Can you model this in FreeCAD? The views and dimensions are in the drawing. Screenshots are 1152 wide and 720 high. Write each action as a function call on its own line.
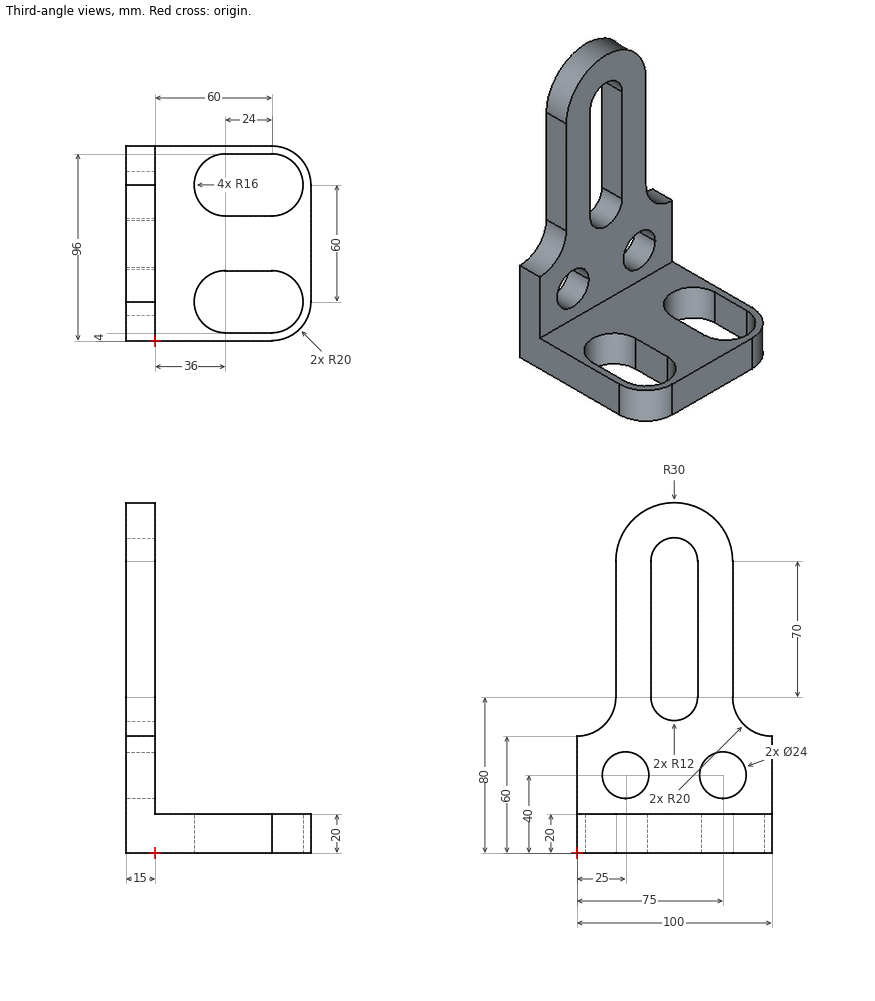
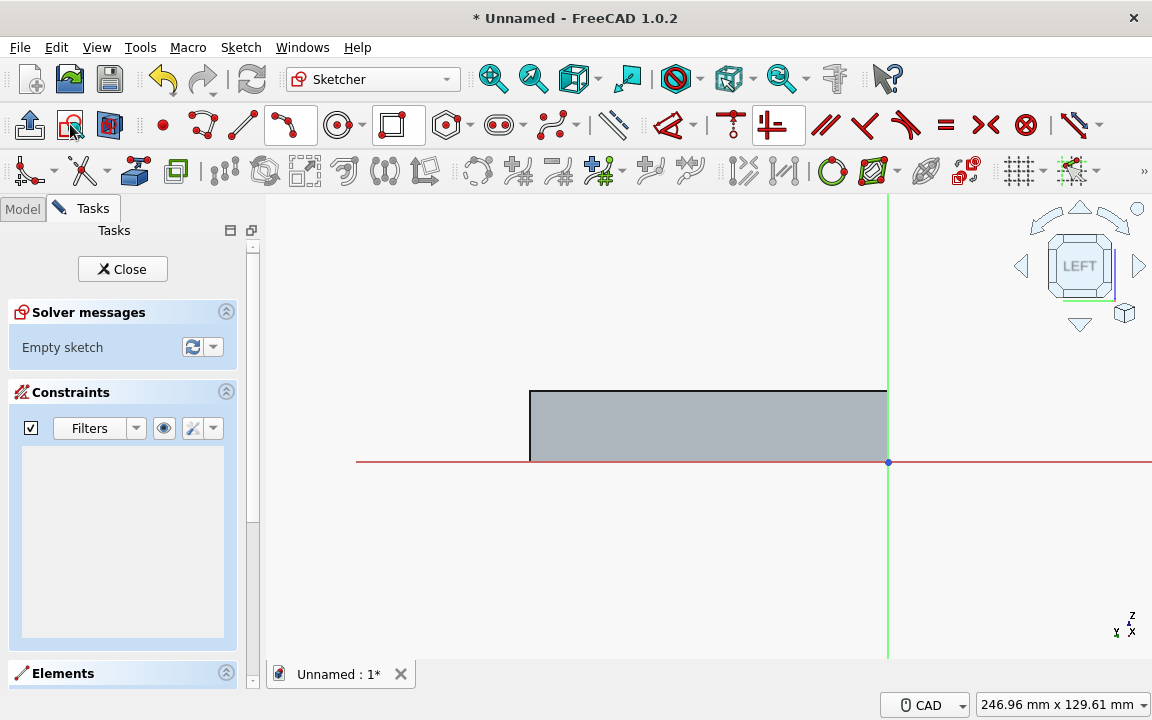
key(g)
key(r)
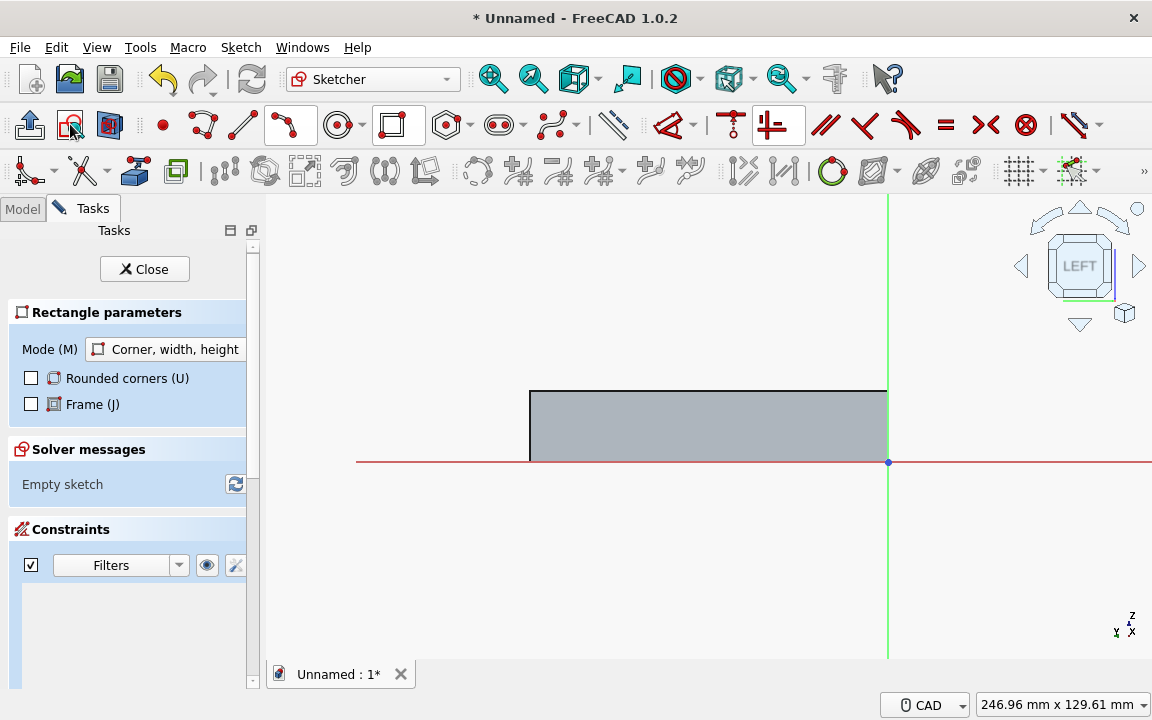
click(888, 462)
move(530, 247)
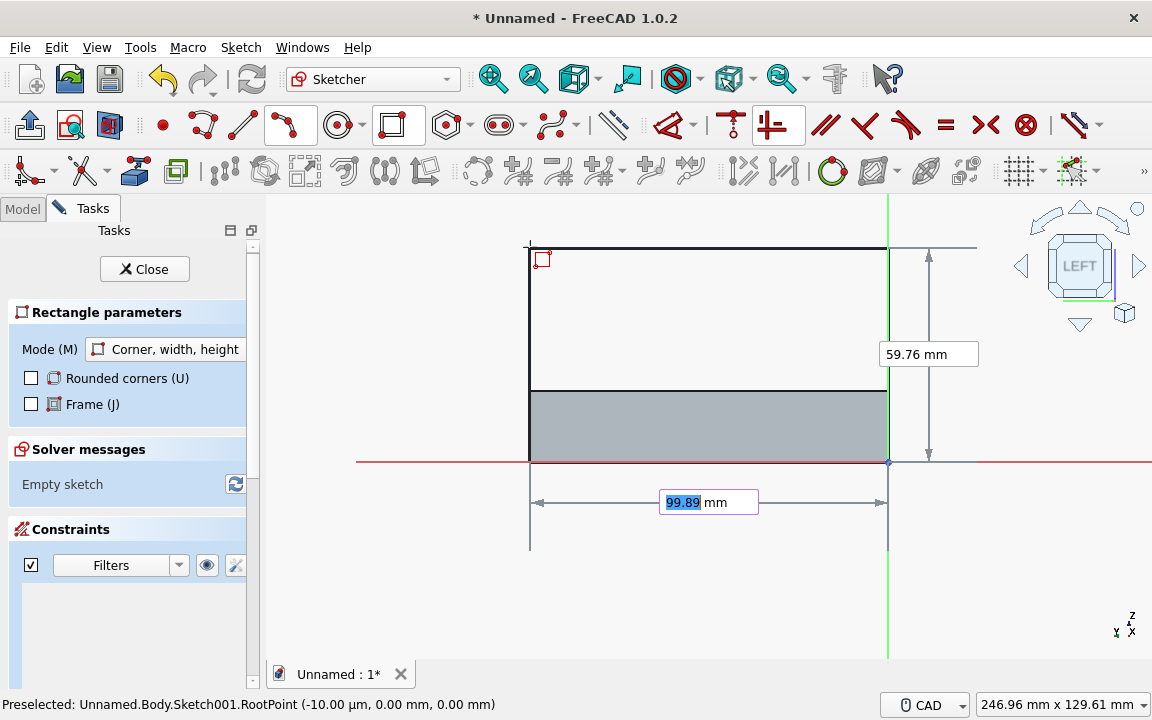
text(100)
key(Tab)
text(60)
key(Return)
key(Escape)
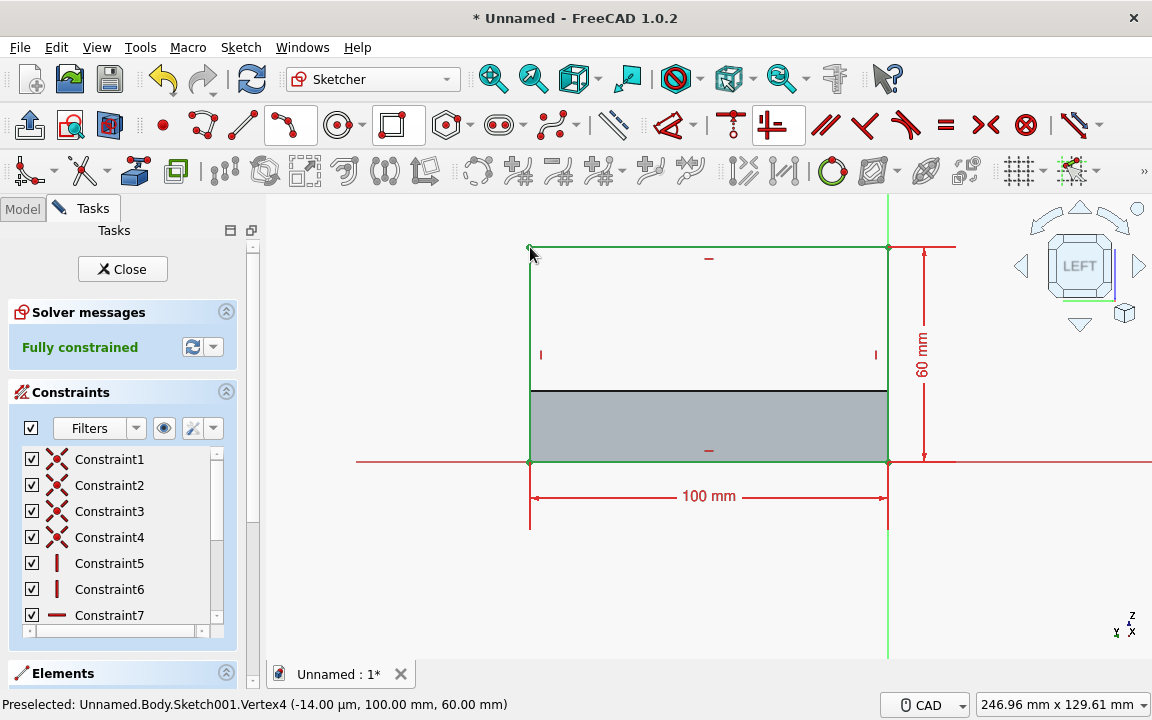
click(123, 269)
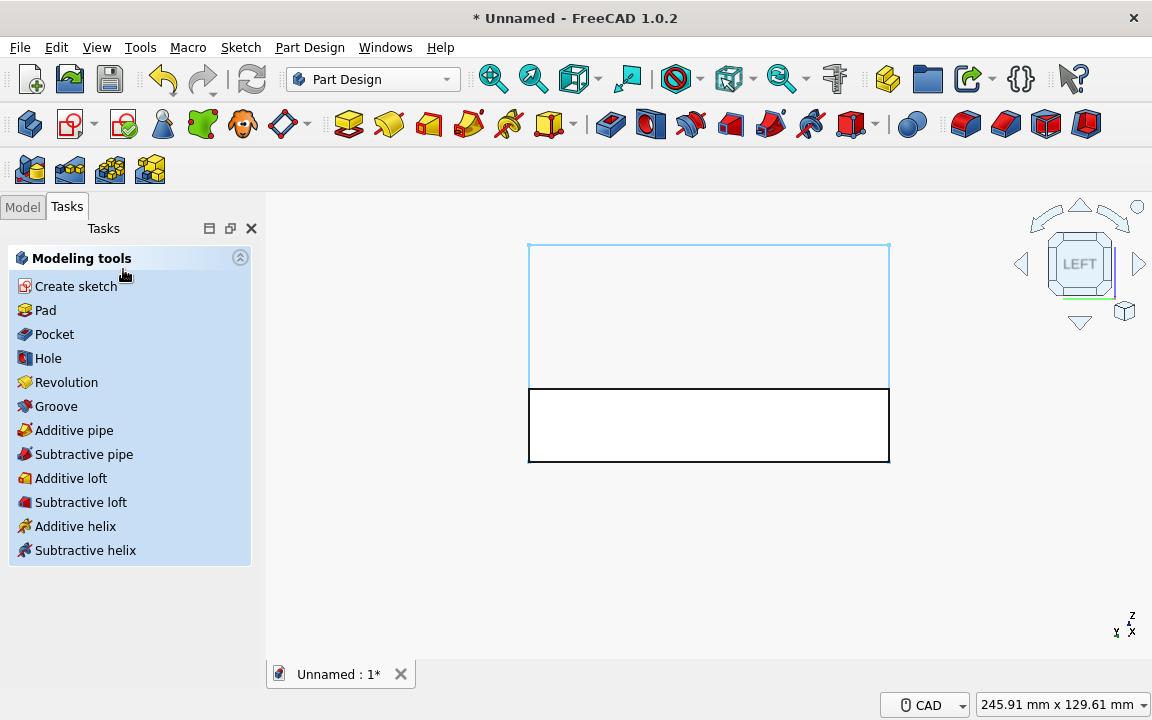
click(350, 124)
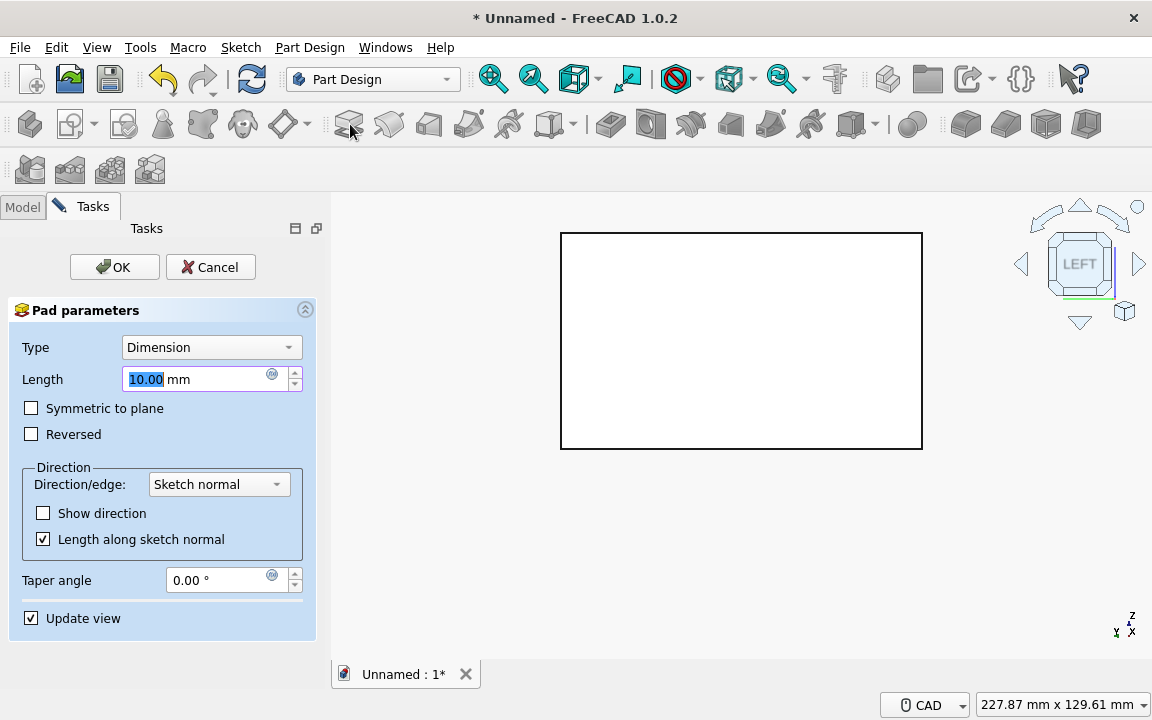
text(15)
key(Tab)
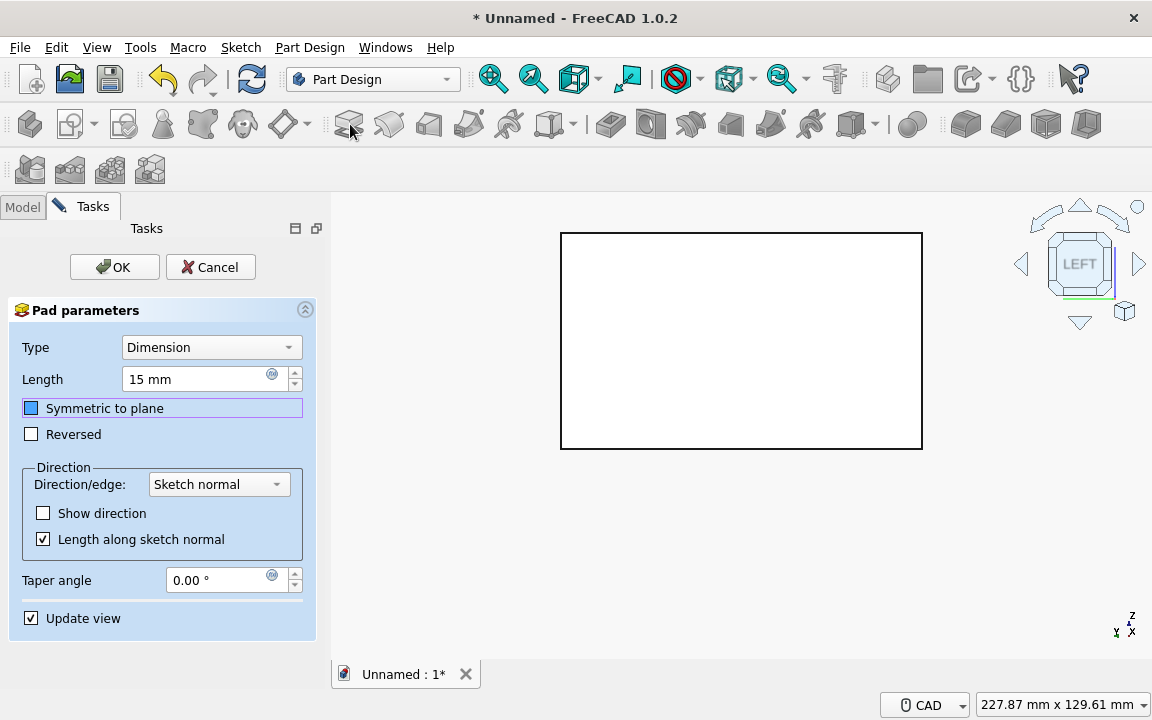
click(115, 267)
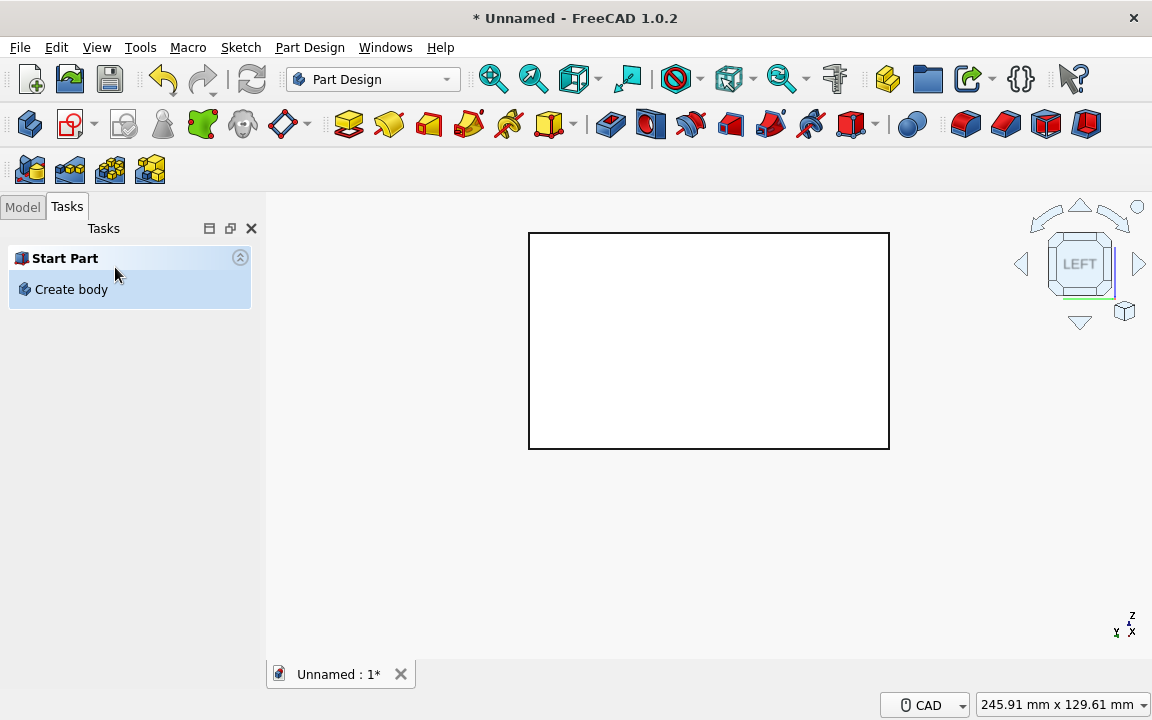
click(658, 340)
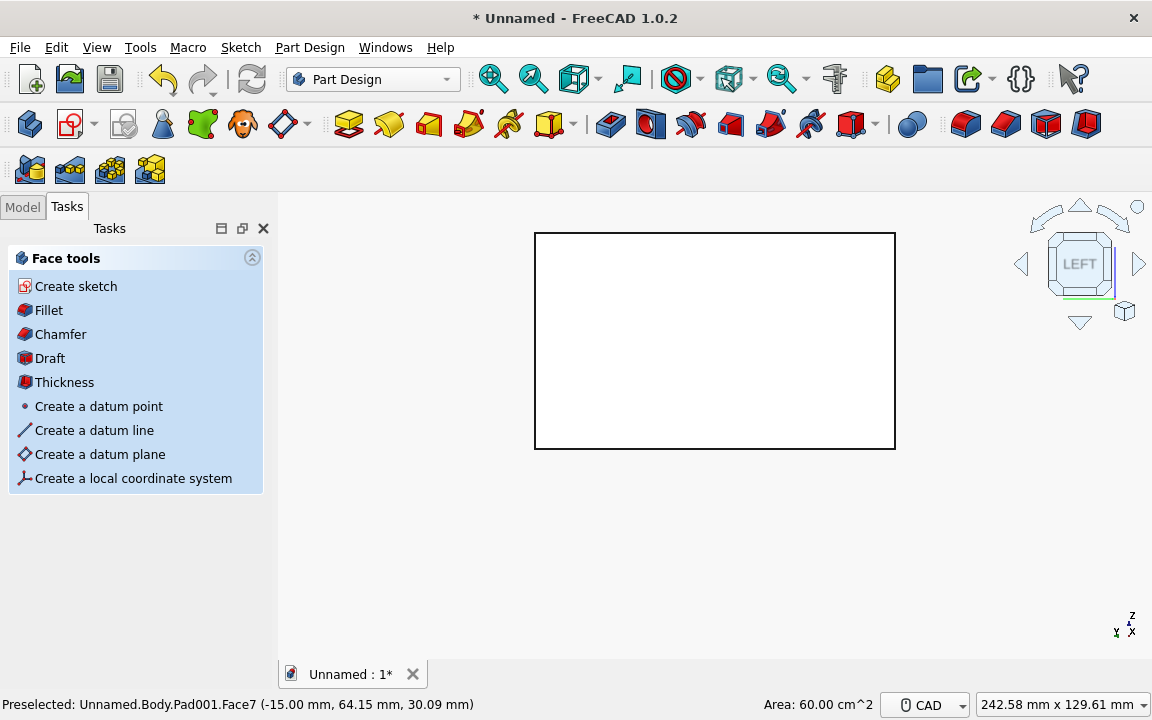
click(70, 124)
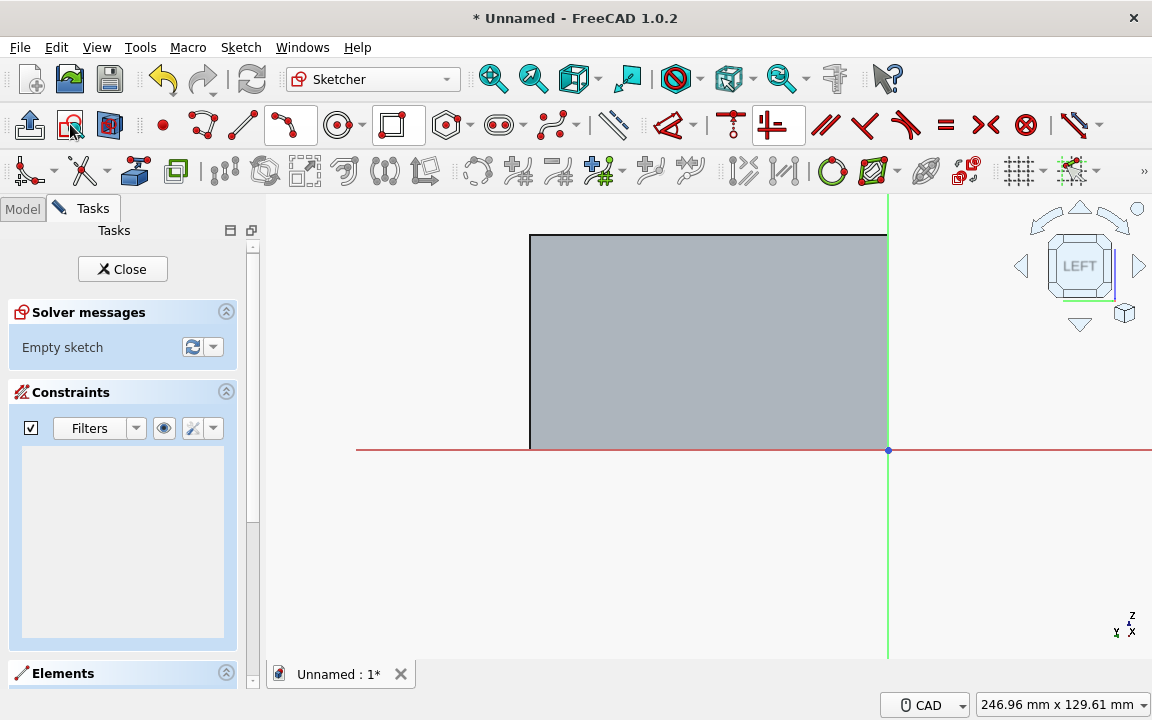
scroll(585, 631, down, 4)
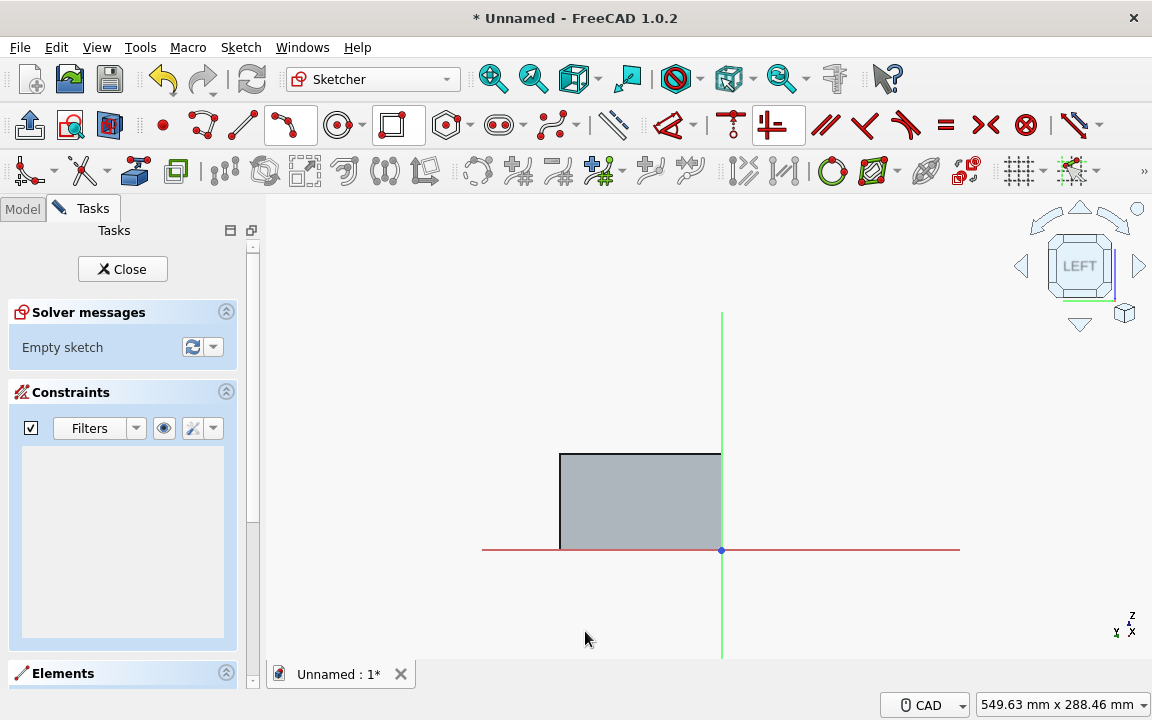
key(g)
key(l)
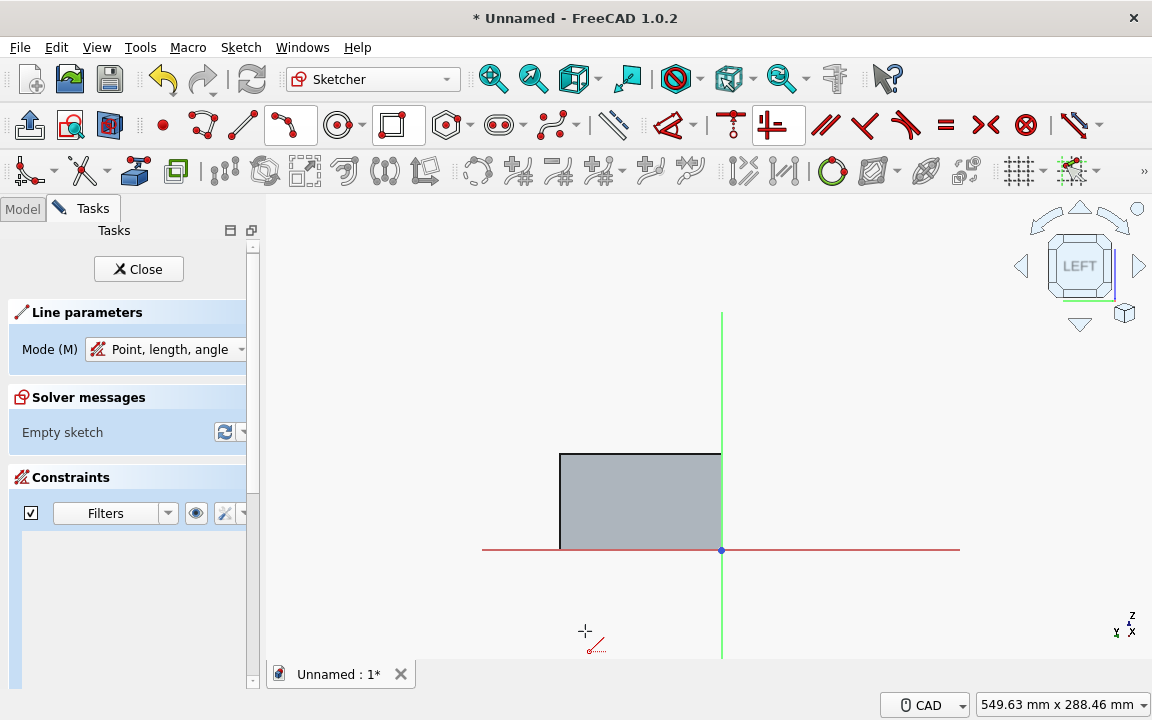
click(593, 309)
click(593, 421)